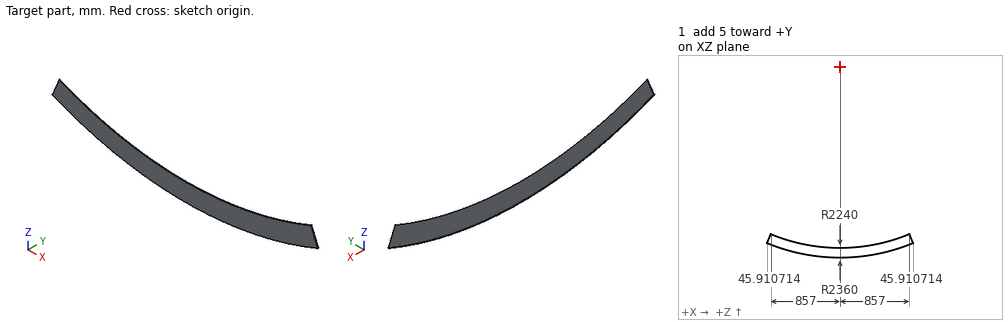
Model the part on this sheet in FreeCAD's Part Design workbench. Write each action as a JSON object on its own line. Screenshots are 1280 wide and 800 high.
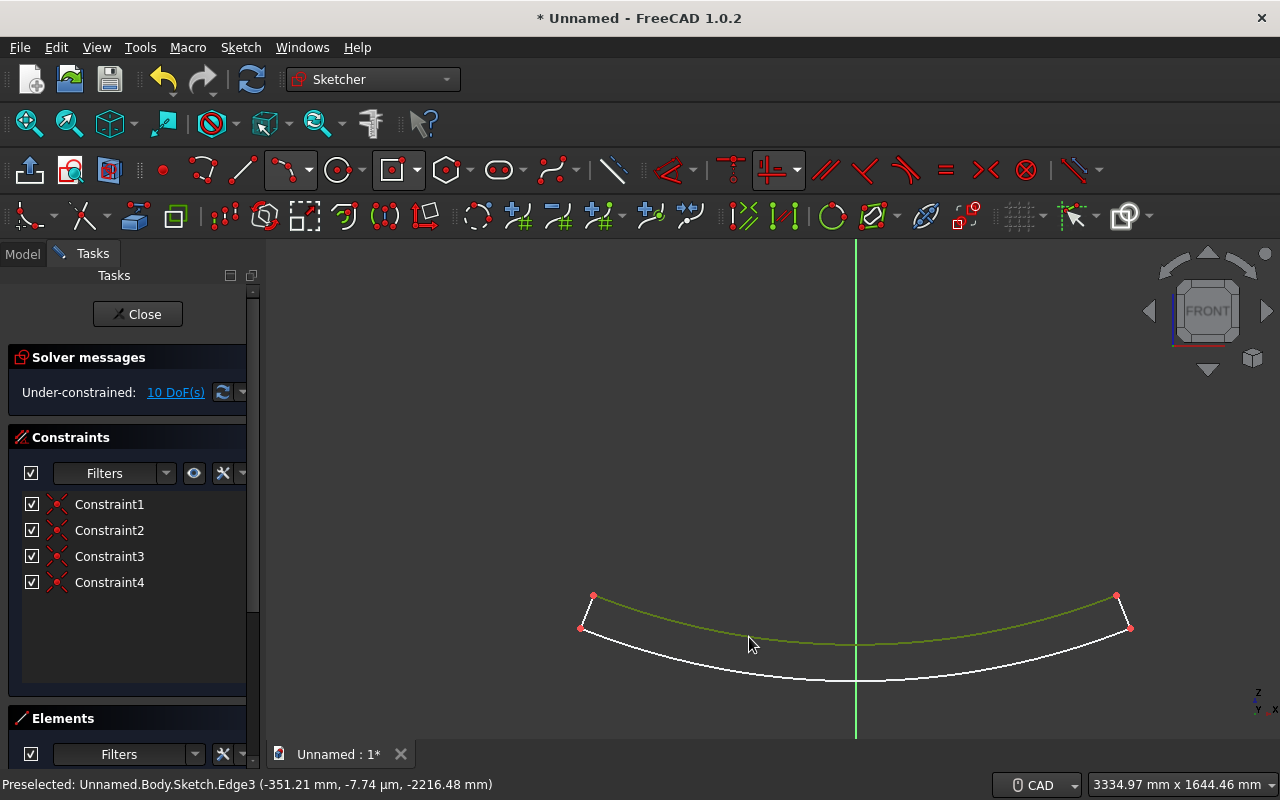
{"action": "left_click", "coordinate": [743, 673]}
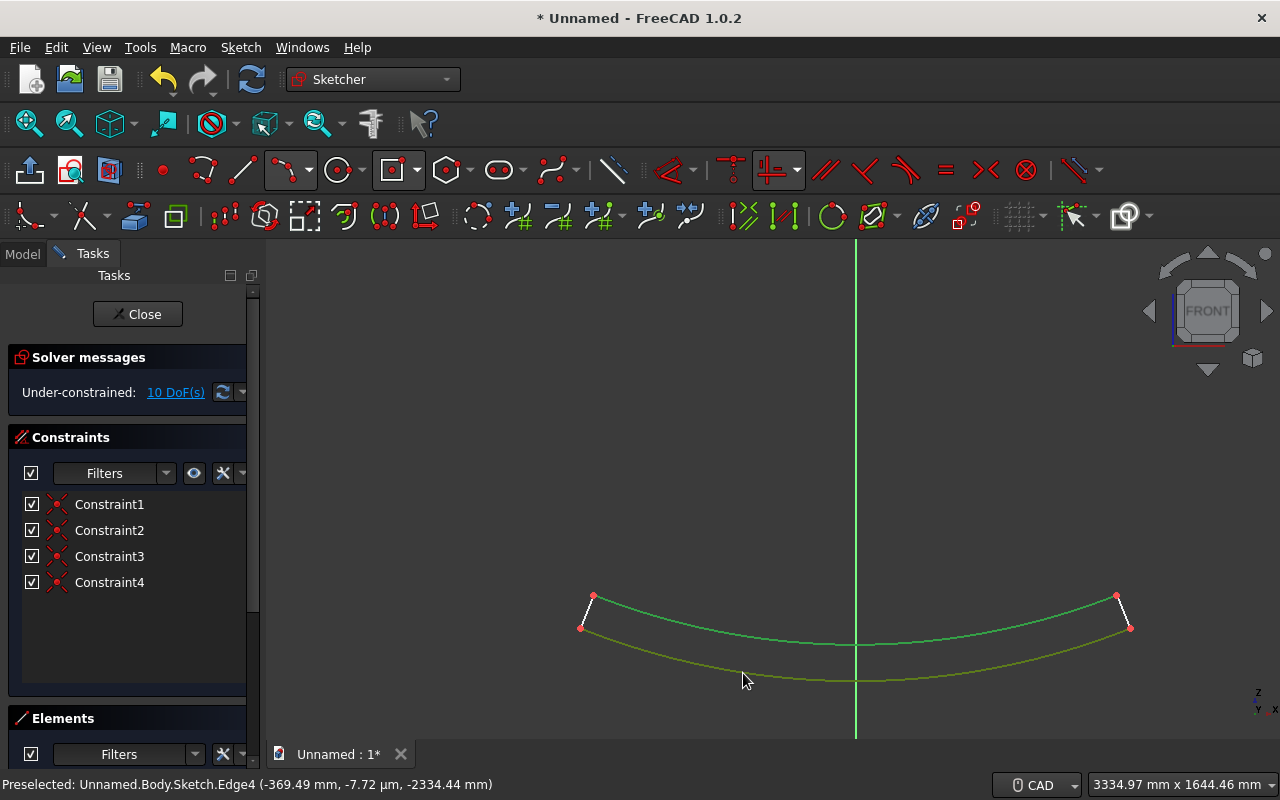
{"action": "left_click", "coordinate": [732, 170]}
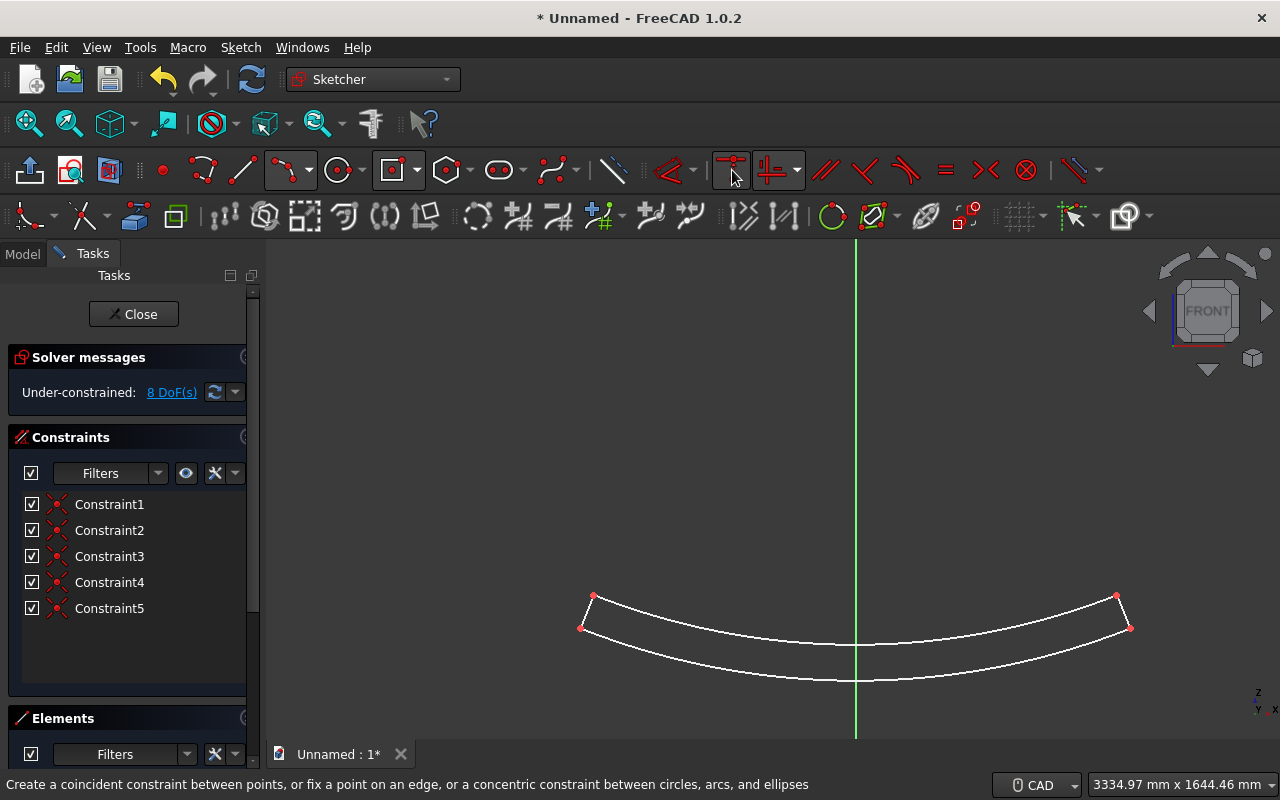
{"action": "scroll", "coordinate": [581, 626], "scroll_direction": "down", "scroll_amount": 4}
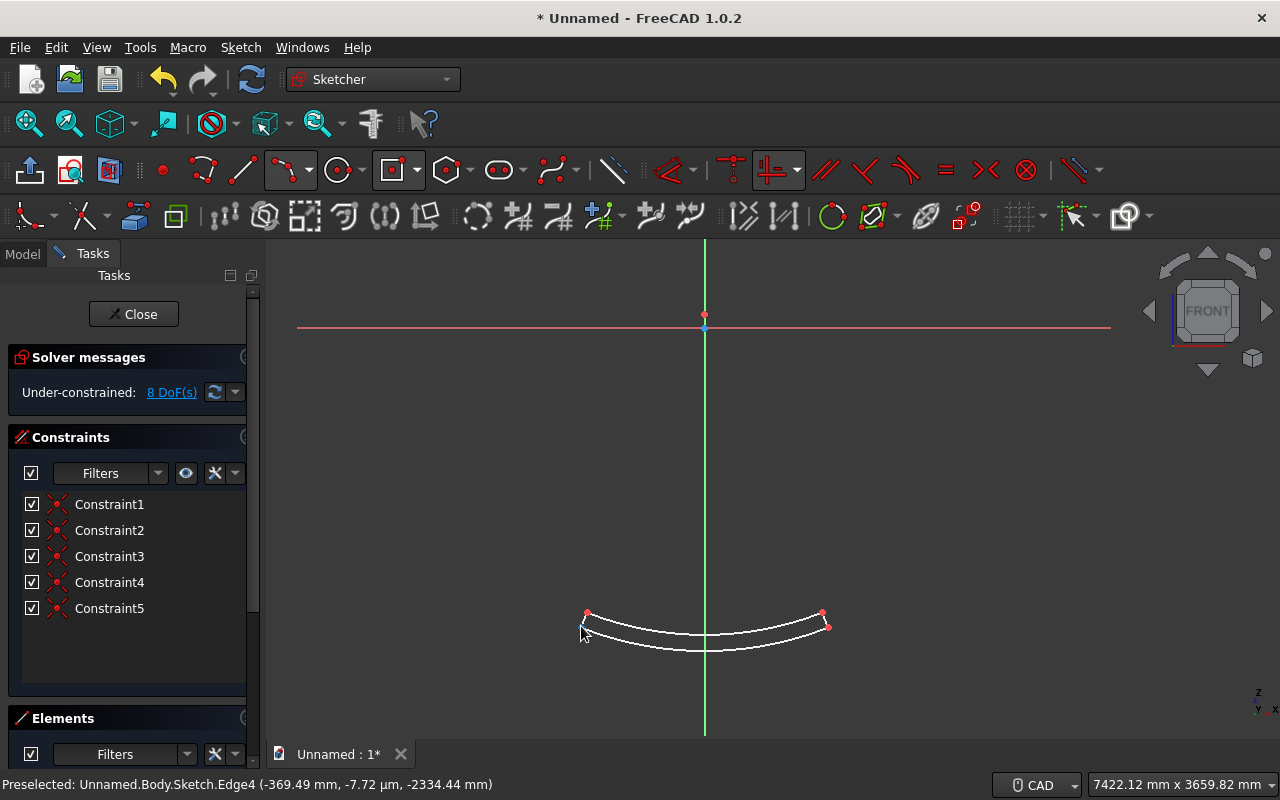
{"action": "left_click_drag", "start_coordinate": [695, 304], "coordinate": [715, 338]}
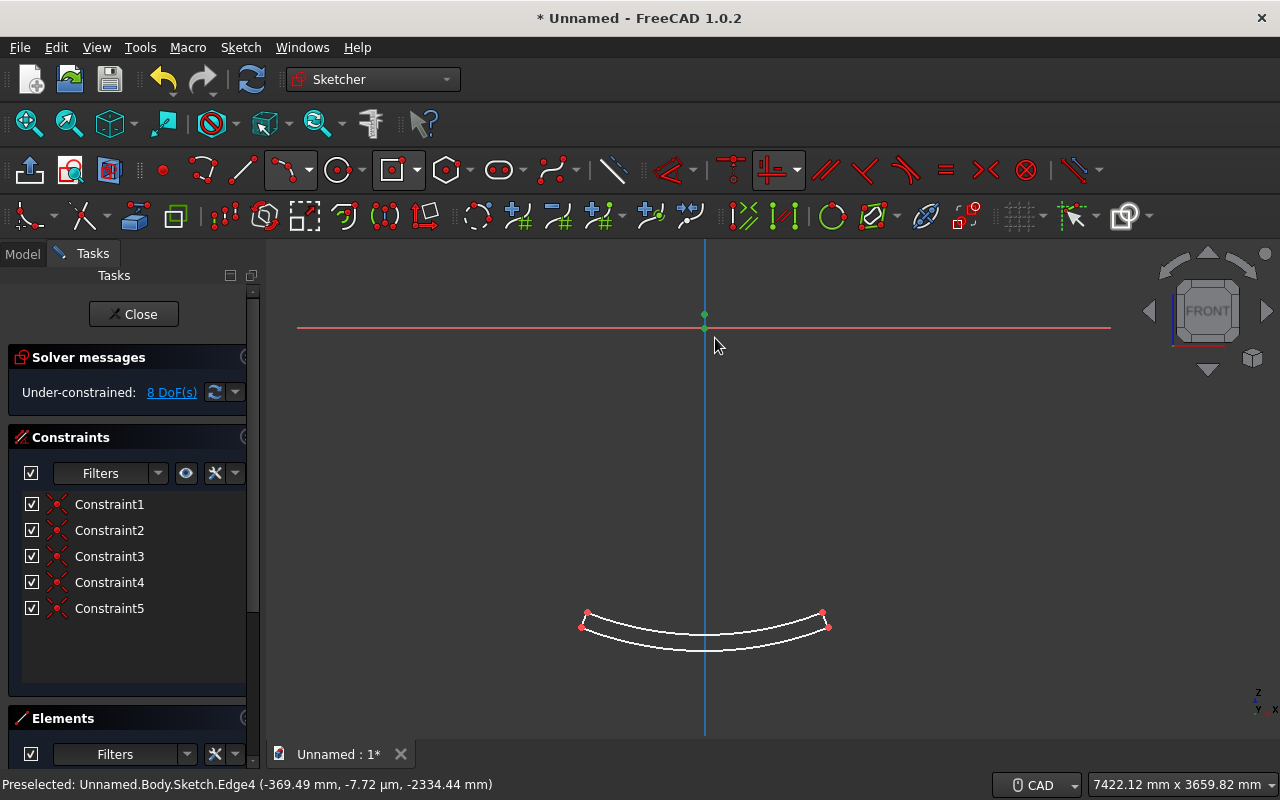
{"action": "left_click", "coordinate": [732, 170]}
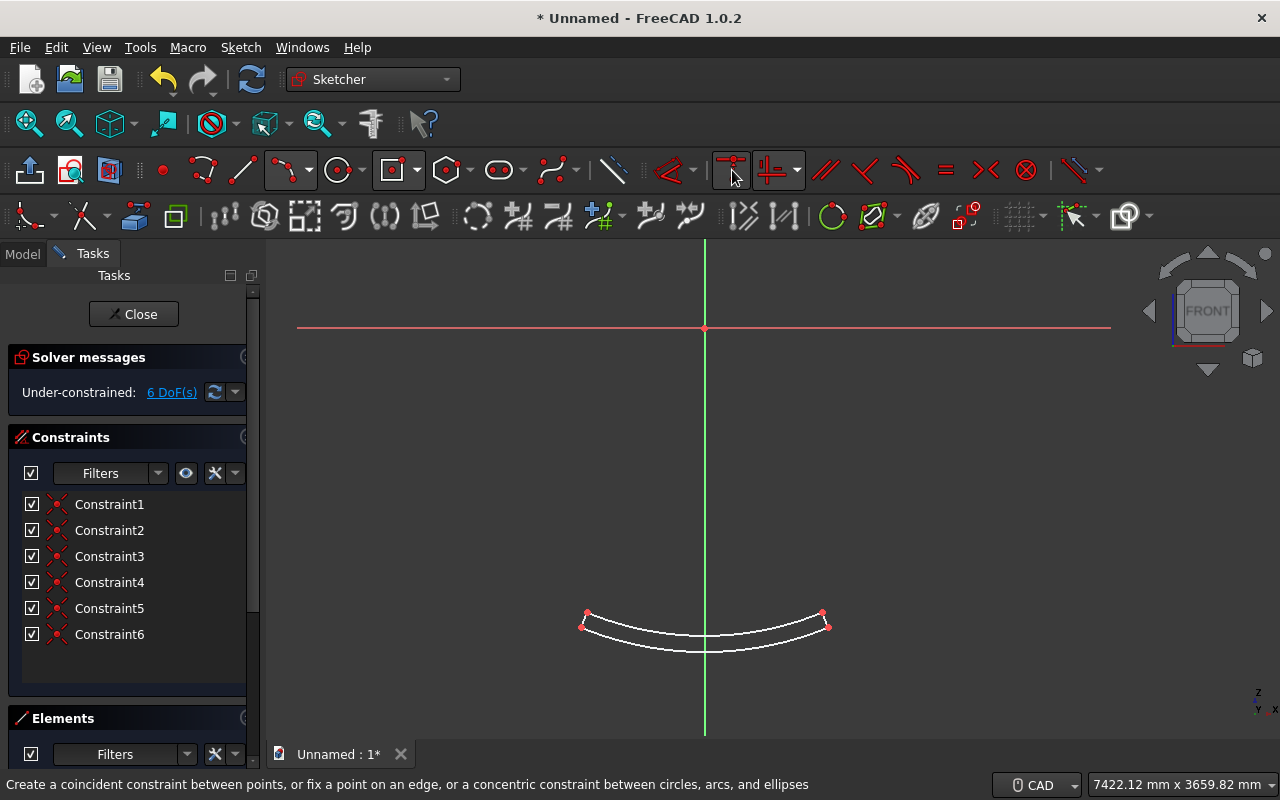
{"action": "left_click", "coordinate": [668, 170]}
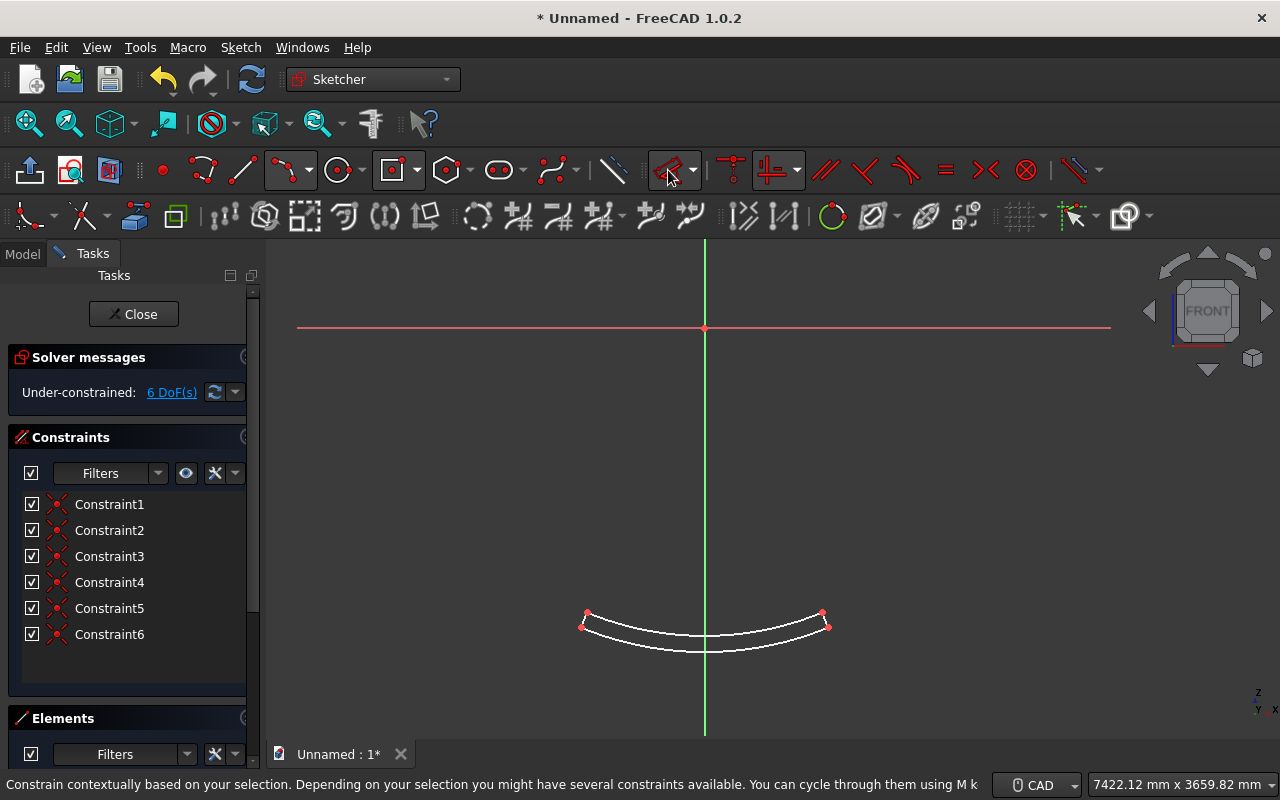
{"action": "left_click", "coordinate": [656, 632]}
{"action": "left_click", "coordinate": [651, 664]}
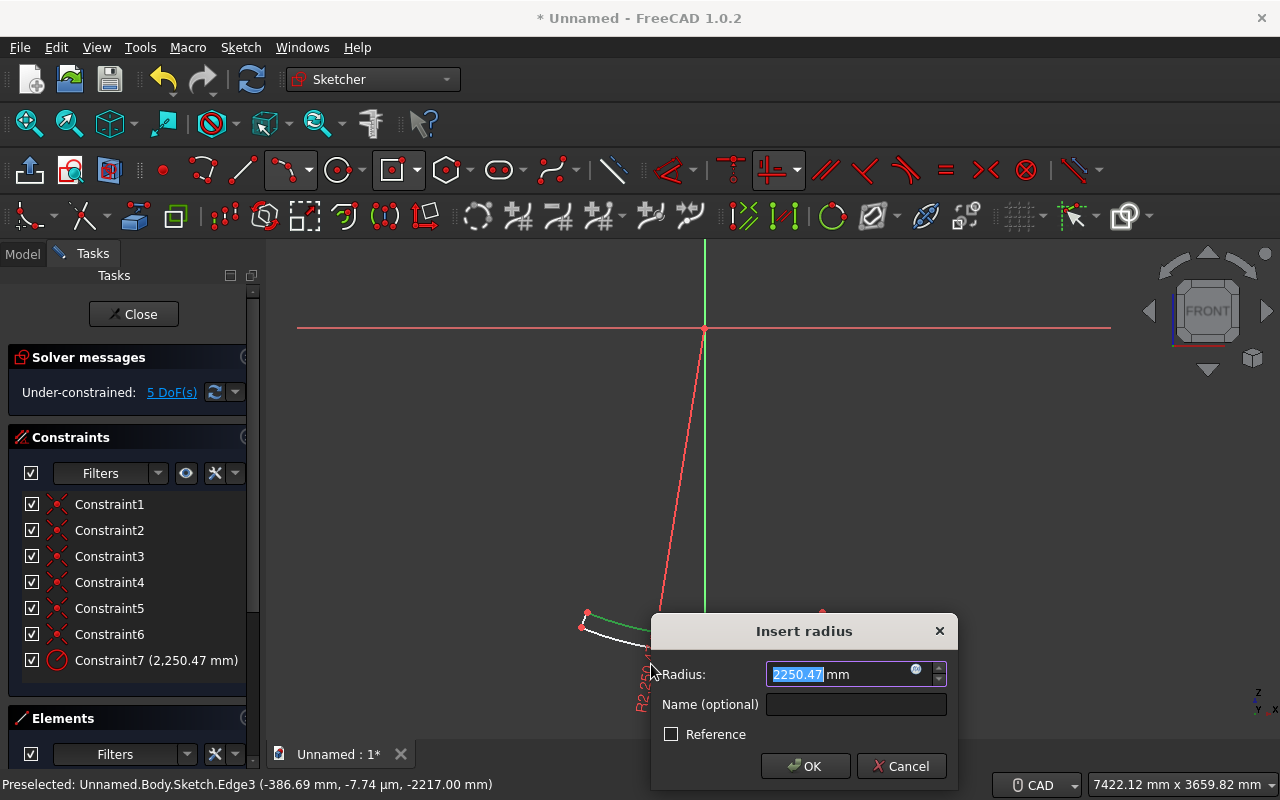
{"action": "type", "text": "2240"}
{"action": "key", "text": "Return"}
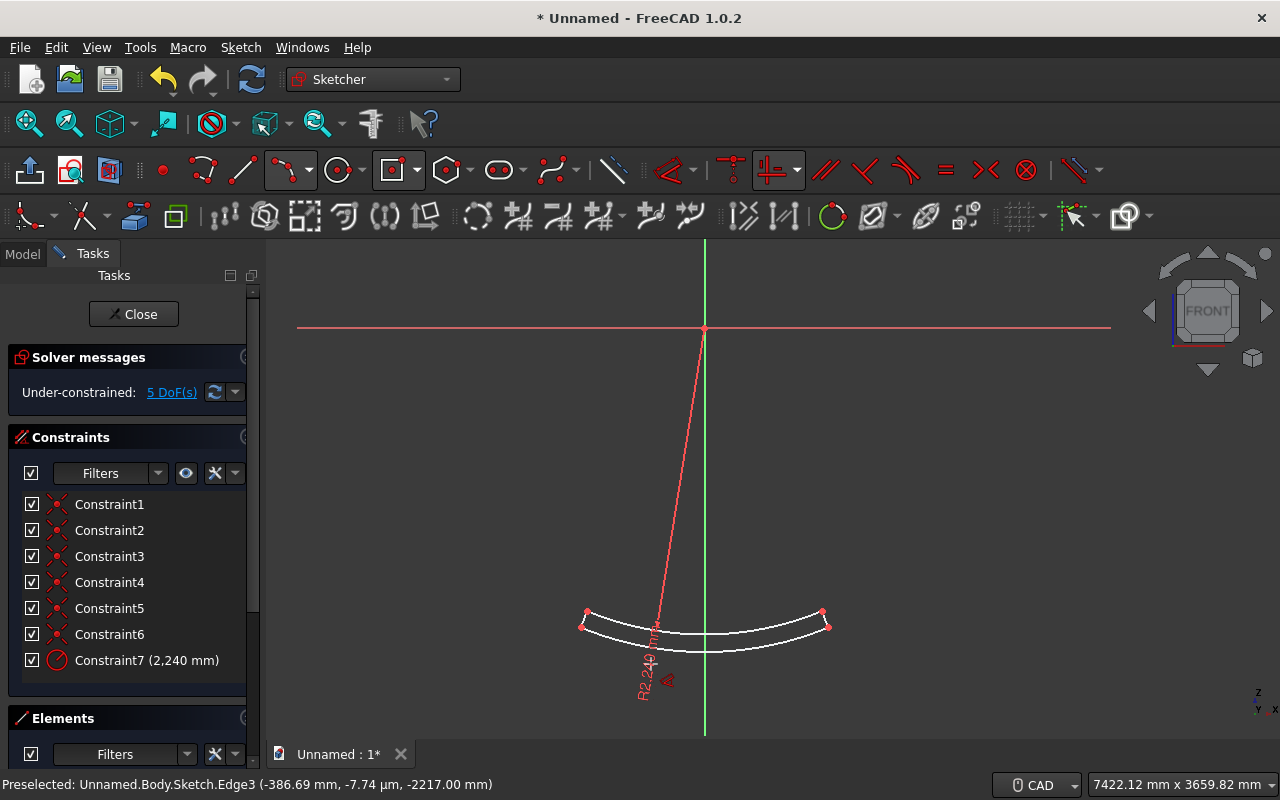
{"action": "left_click", "coordinate": [654, 648]}
{"action": "left_click", "coordinate": [487, 610]}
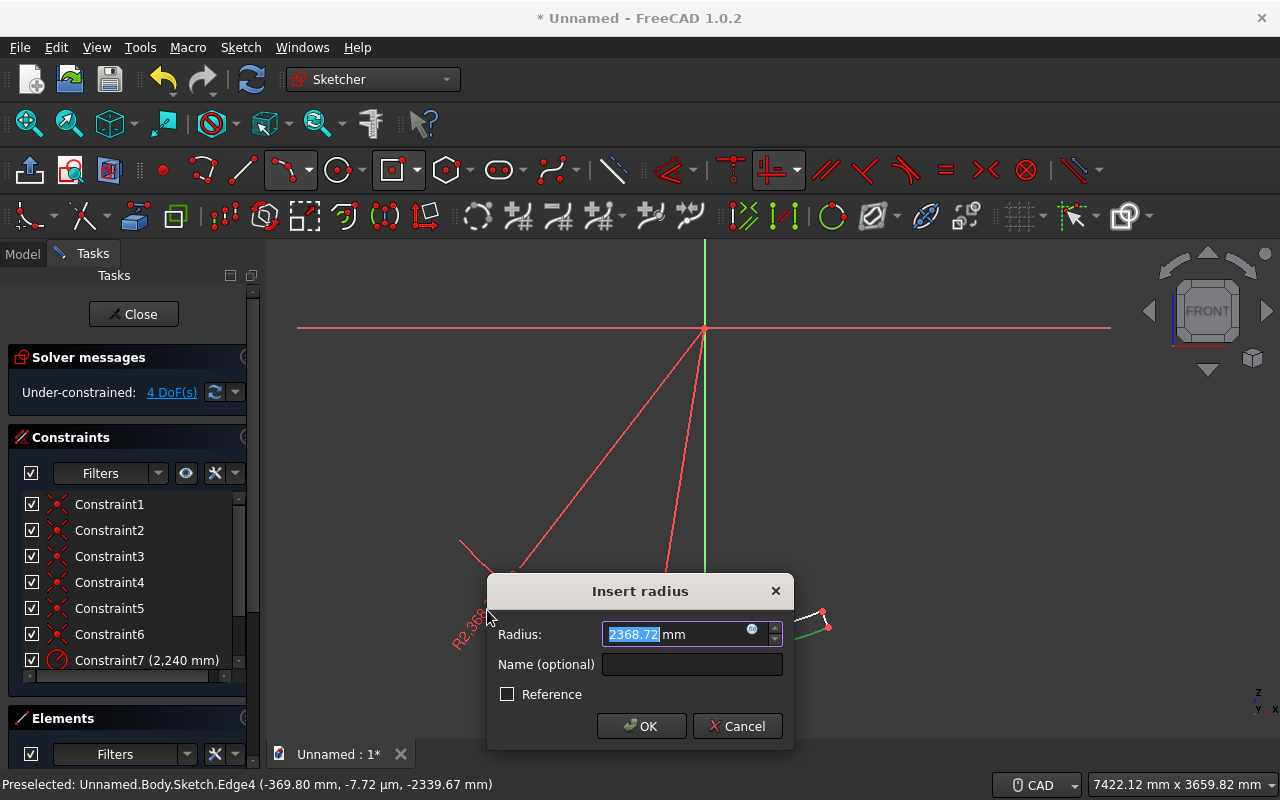
{"action": "type", "text": "2360"}
{"action": "key", "text": "Return"}